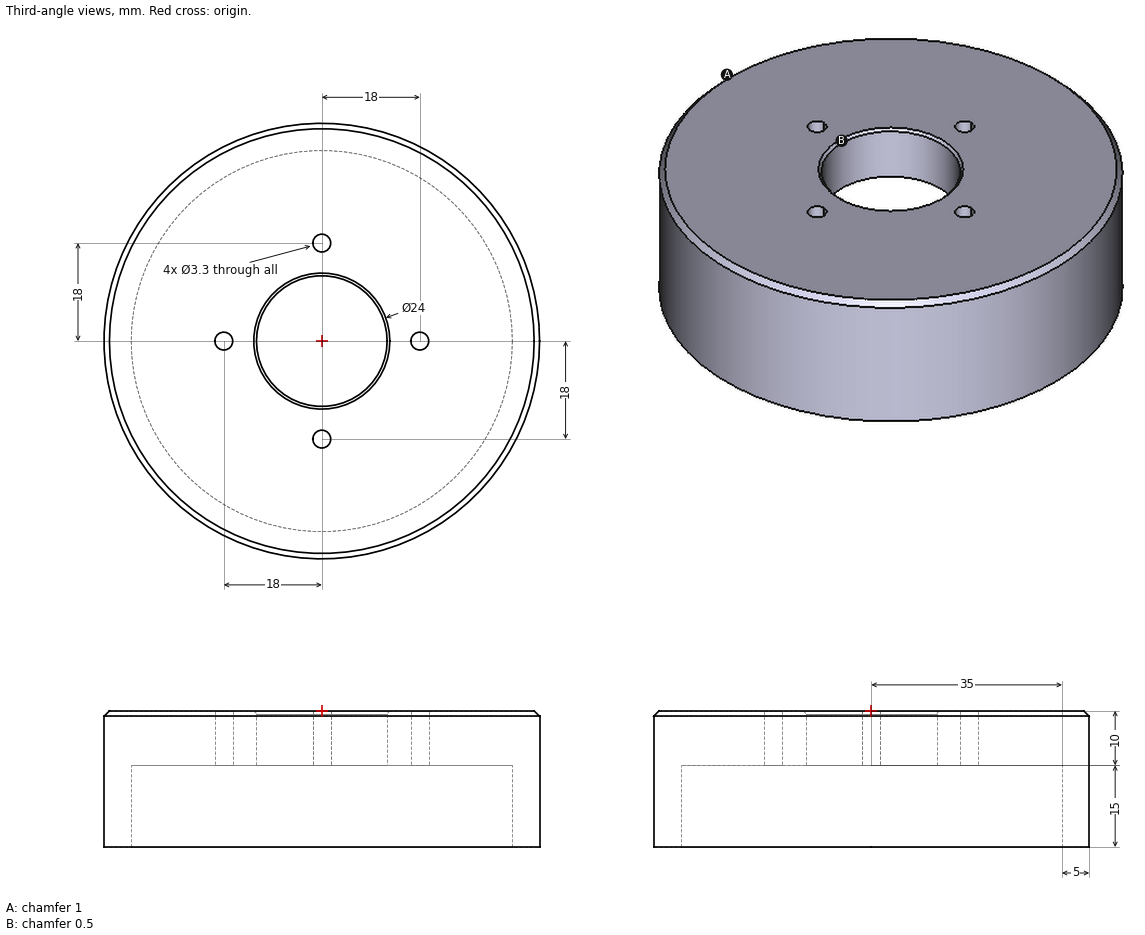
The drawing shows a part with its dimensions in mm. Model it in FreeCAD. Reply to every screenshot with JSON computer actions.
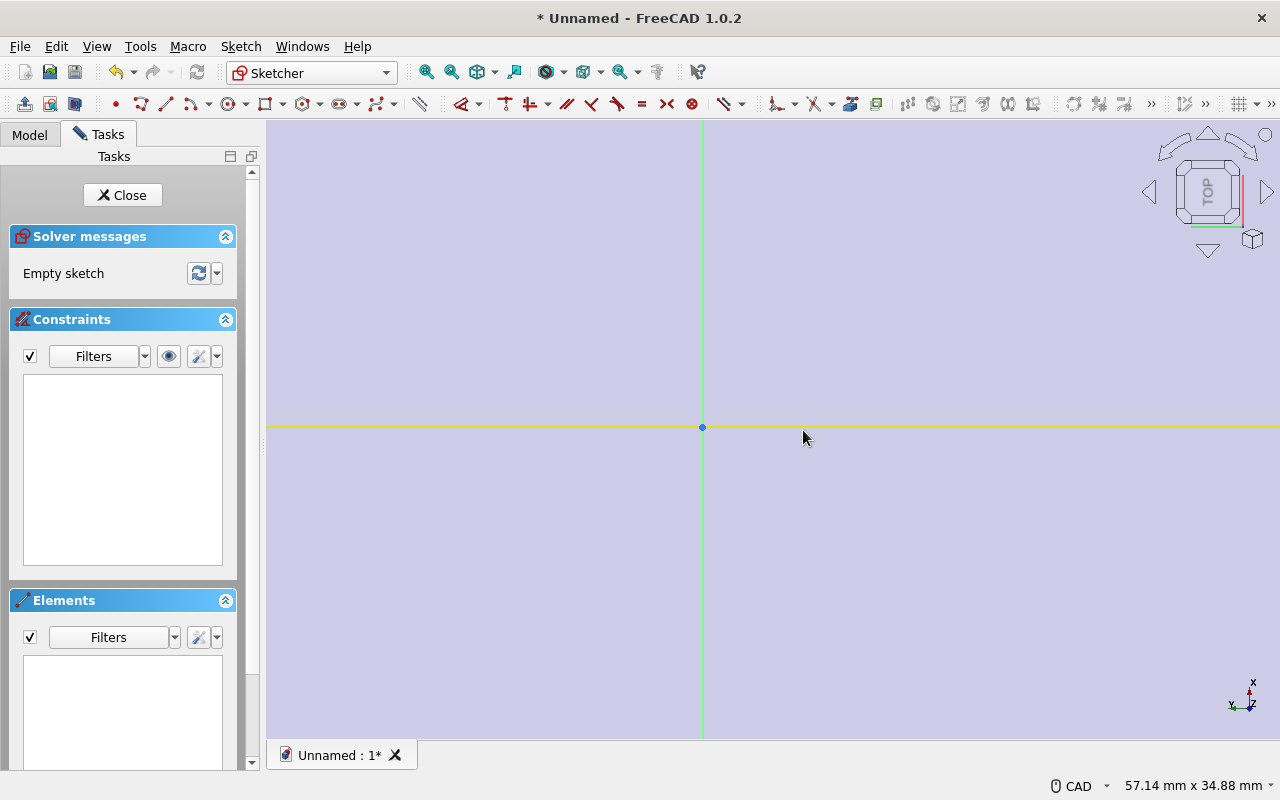
{"action": "key", "text": "g c"}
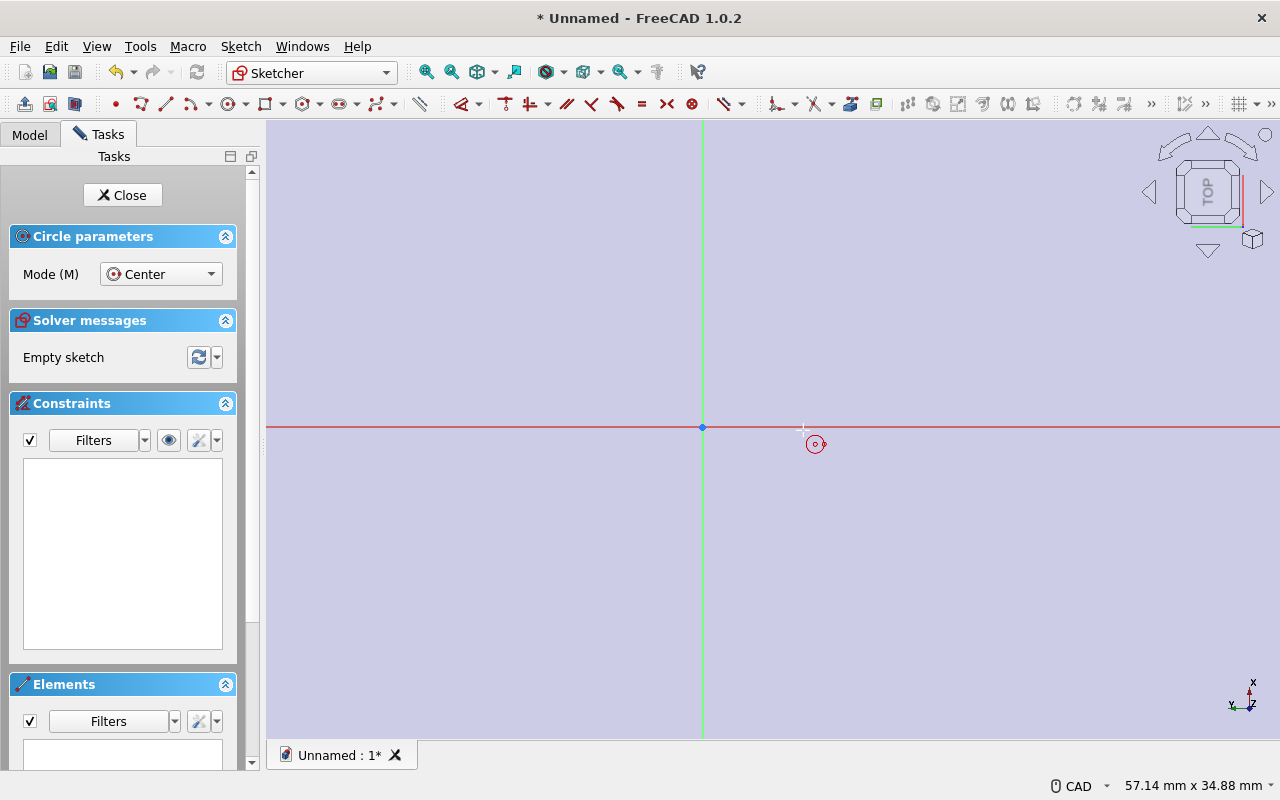
{"action": "left_click", "coordinate": [703, 427]}
{"action": "mouse_move", "coordinate": [853, 277]}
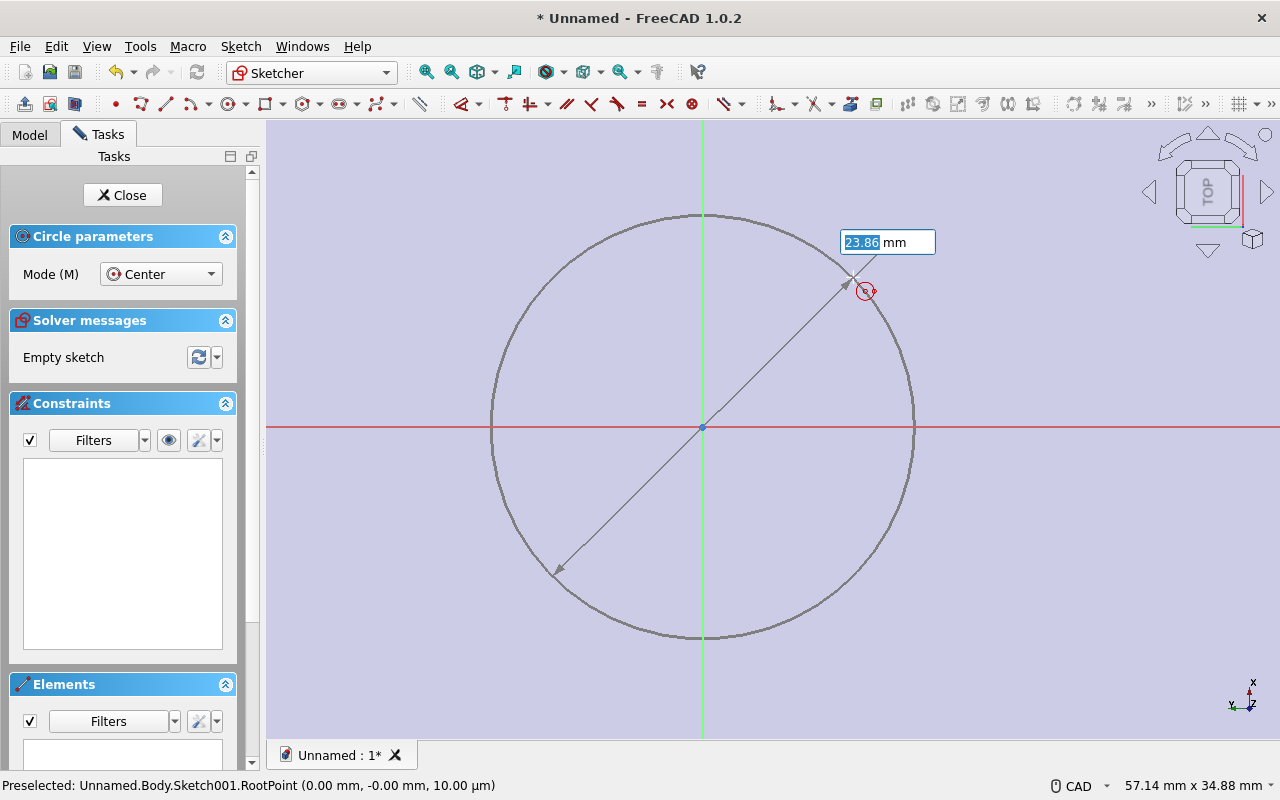
{"action": "type", "text": "24"}
{"action": "key", "text": "Return"}
{"action": "key", "text": "Escape"}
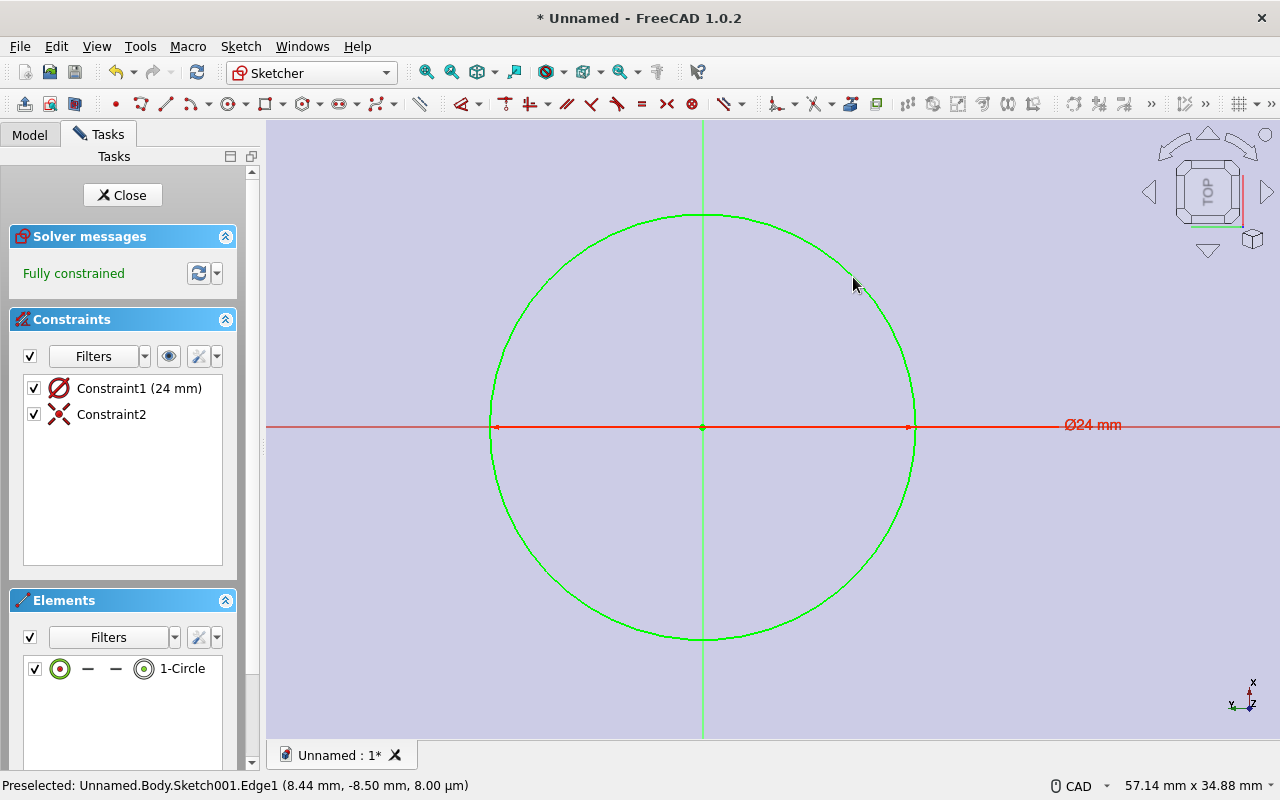
{"action": "left_click", "coordinate": [123, 195]}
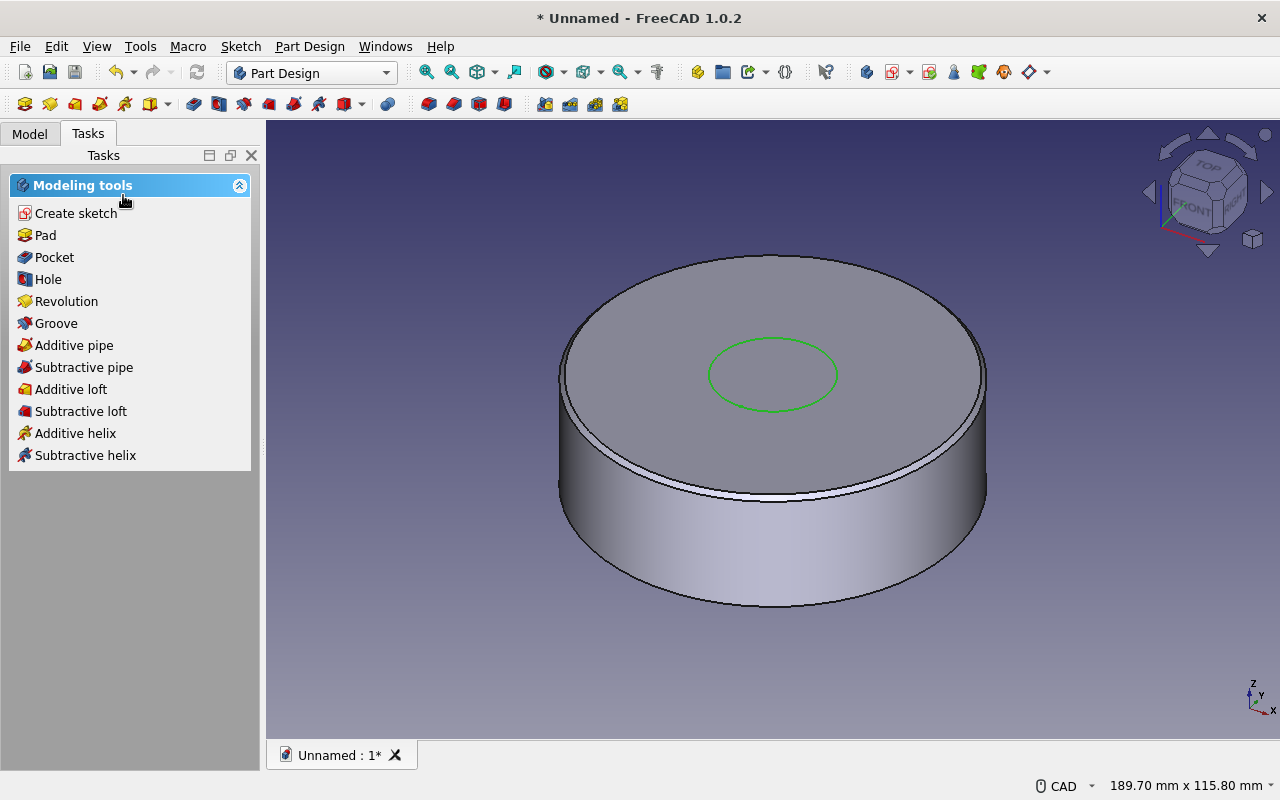
{"action": "left_click", "coordinate": [194, 104]}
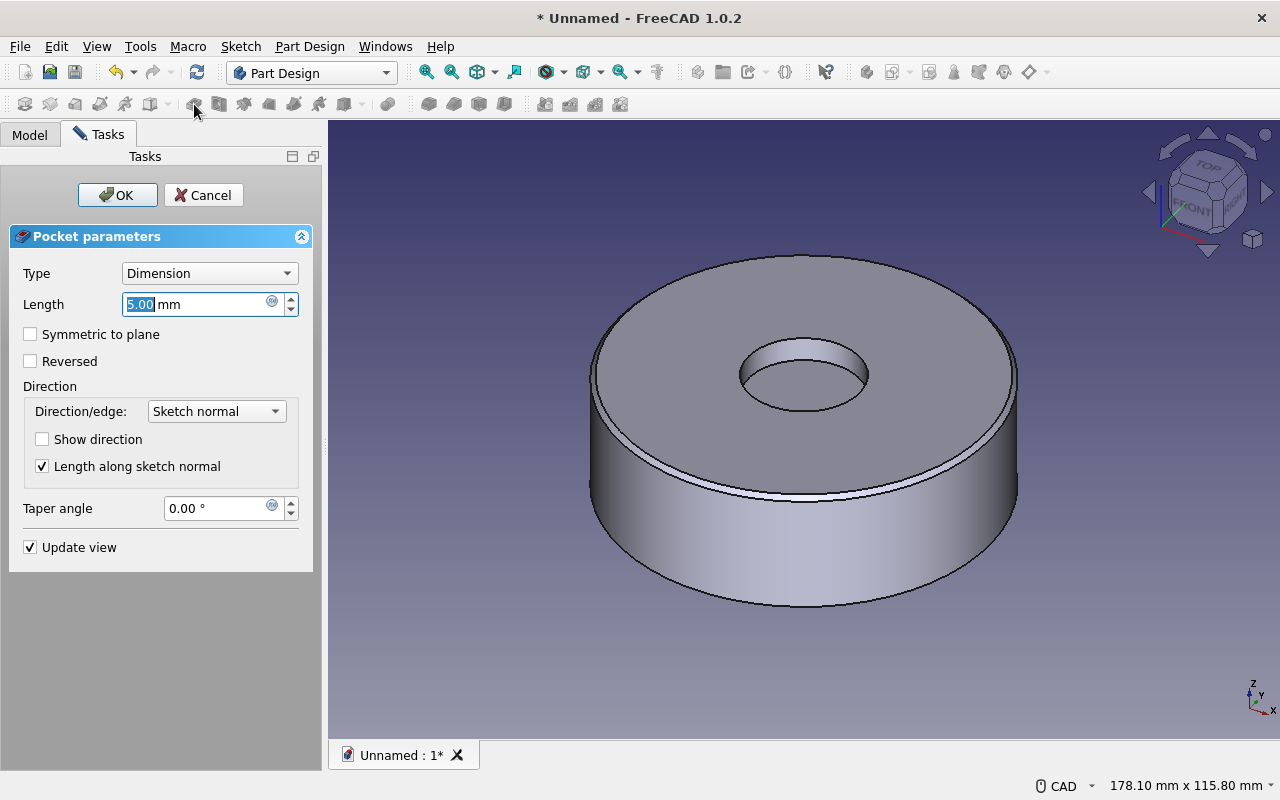
{"action": "left_click", "coordinate": [210, 274]}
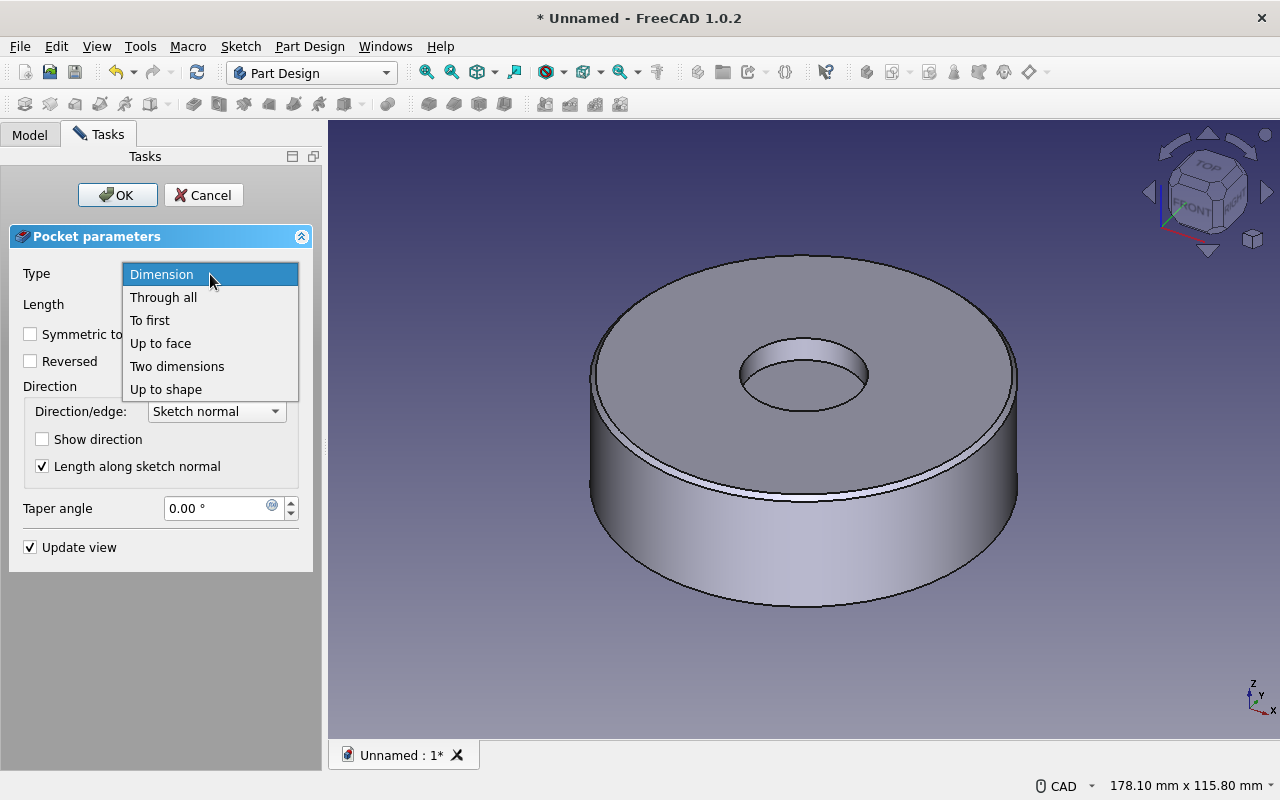
{"action": "left_click", "coordinate": [208, 298]}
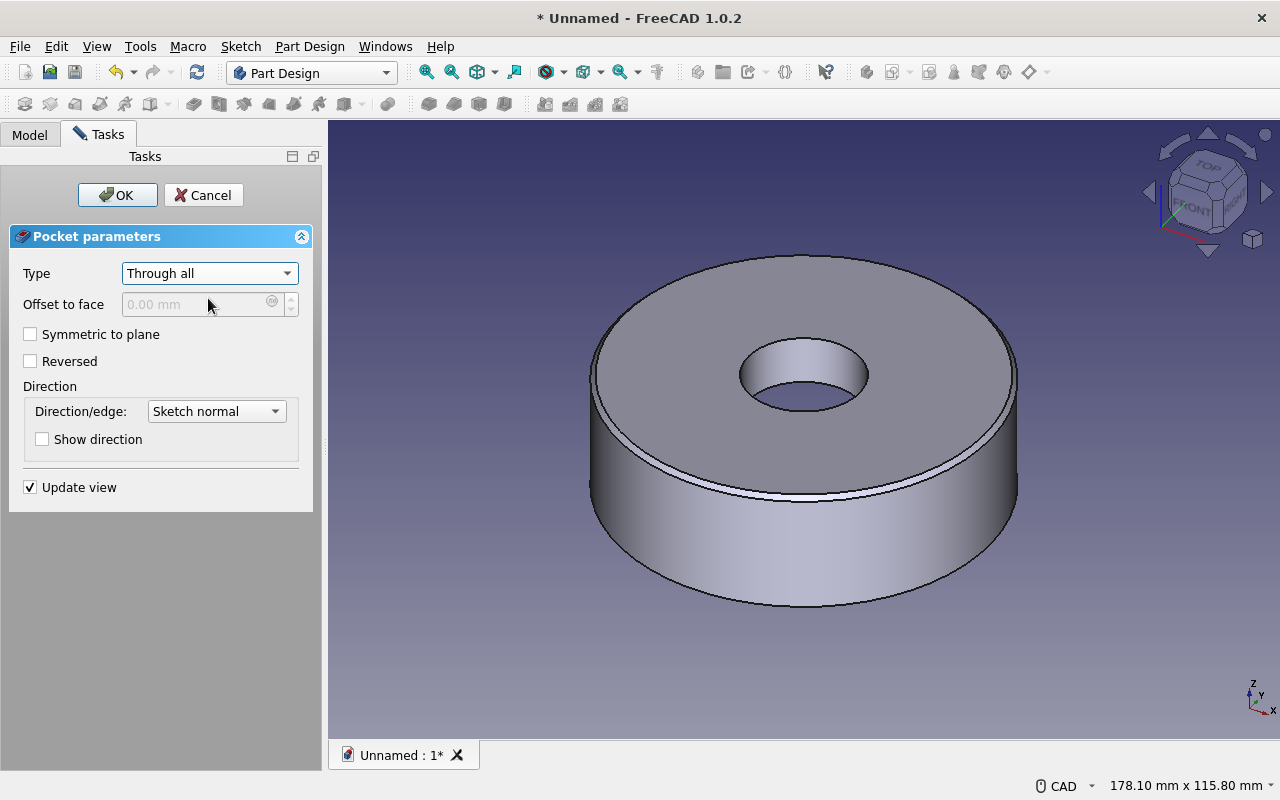
{"action": "left_click", "coordinate": [118, 195]}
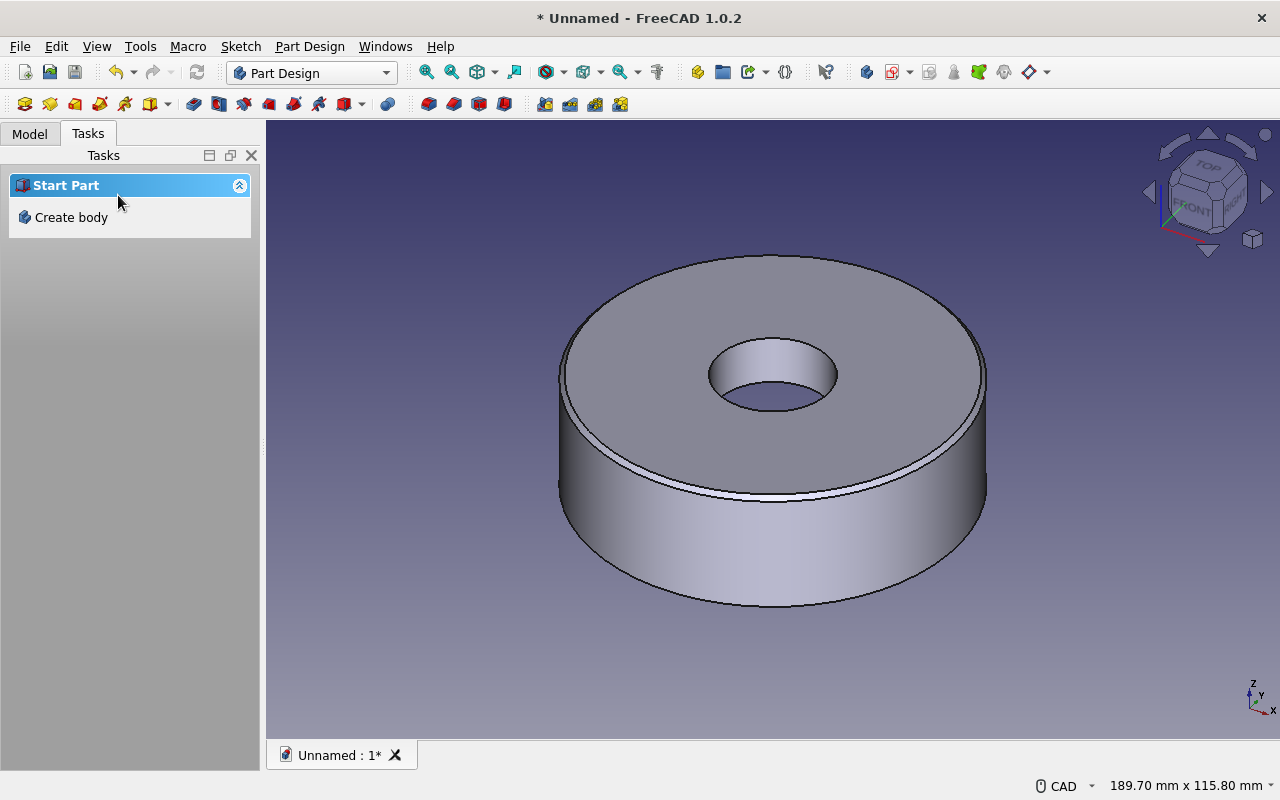
{"action": "left_click", "coordinate": [765, 450]}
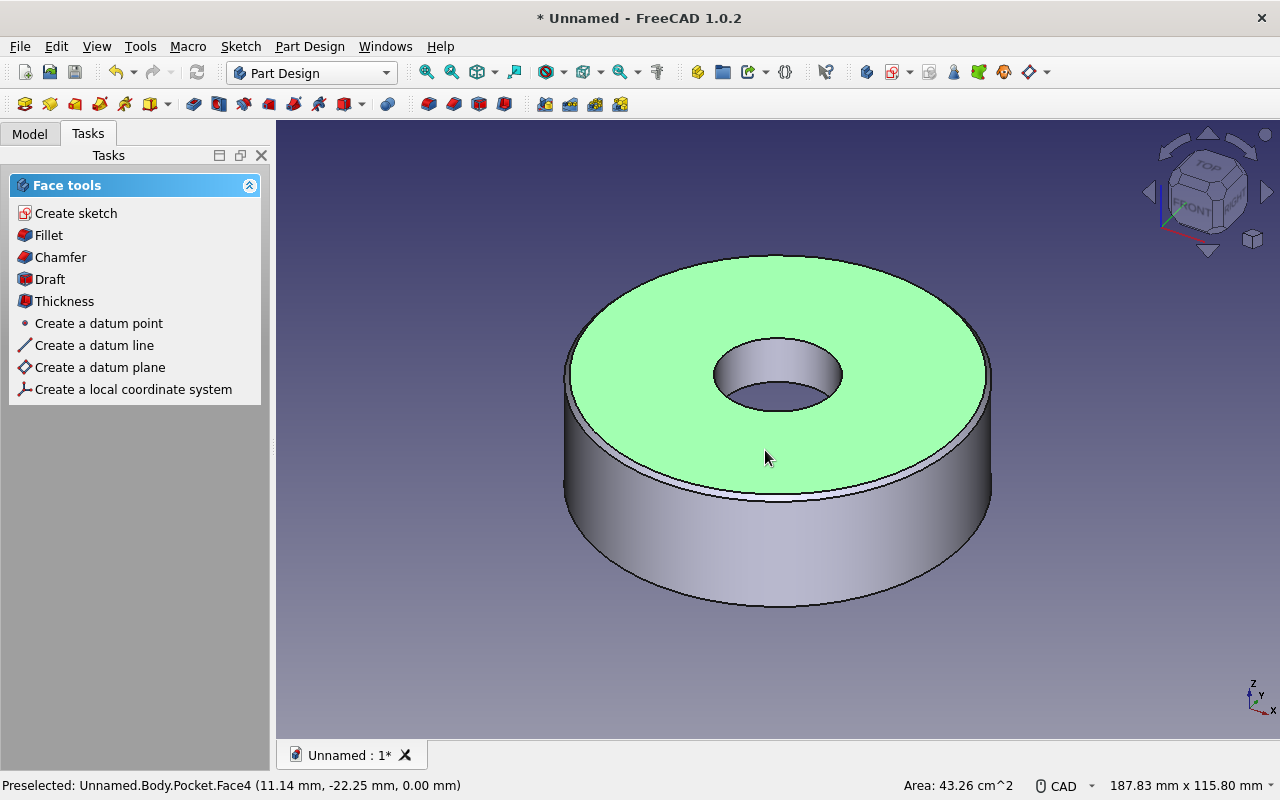
{"action": "left_click", "coordinate": [892, 72]}